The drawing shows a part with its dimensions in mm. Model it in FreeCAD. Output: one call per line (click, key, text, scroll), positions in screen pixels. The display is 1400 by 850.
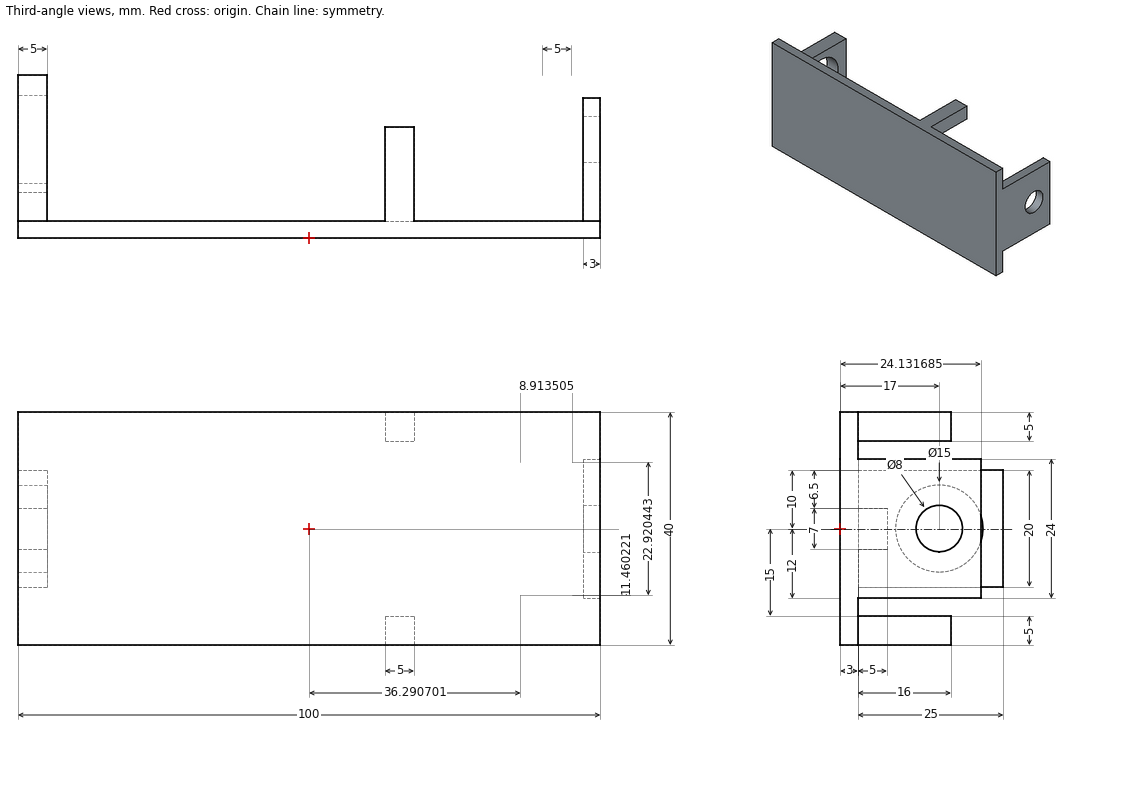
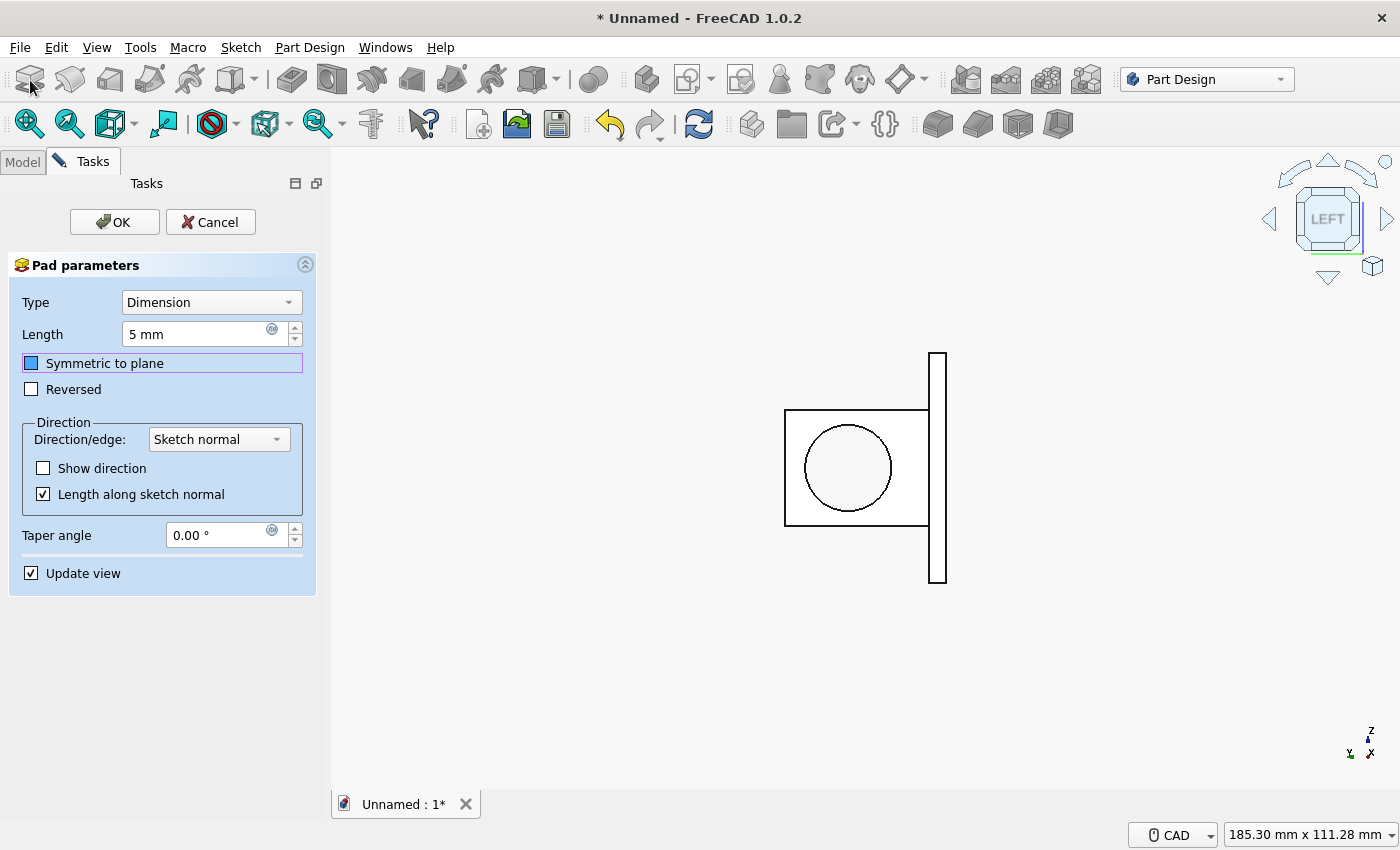
click(30, 389)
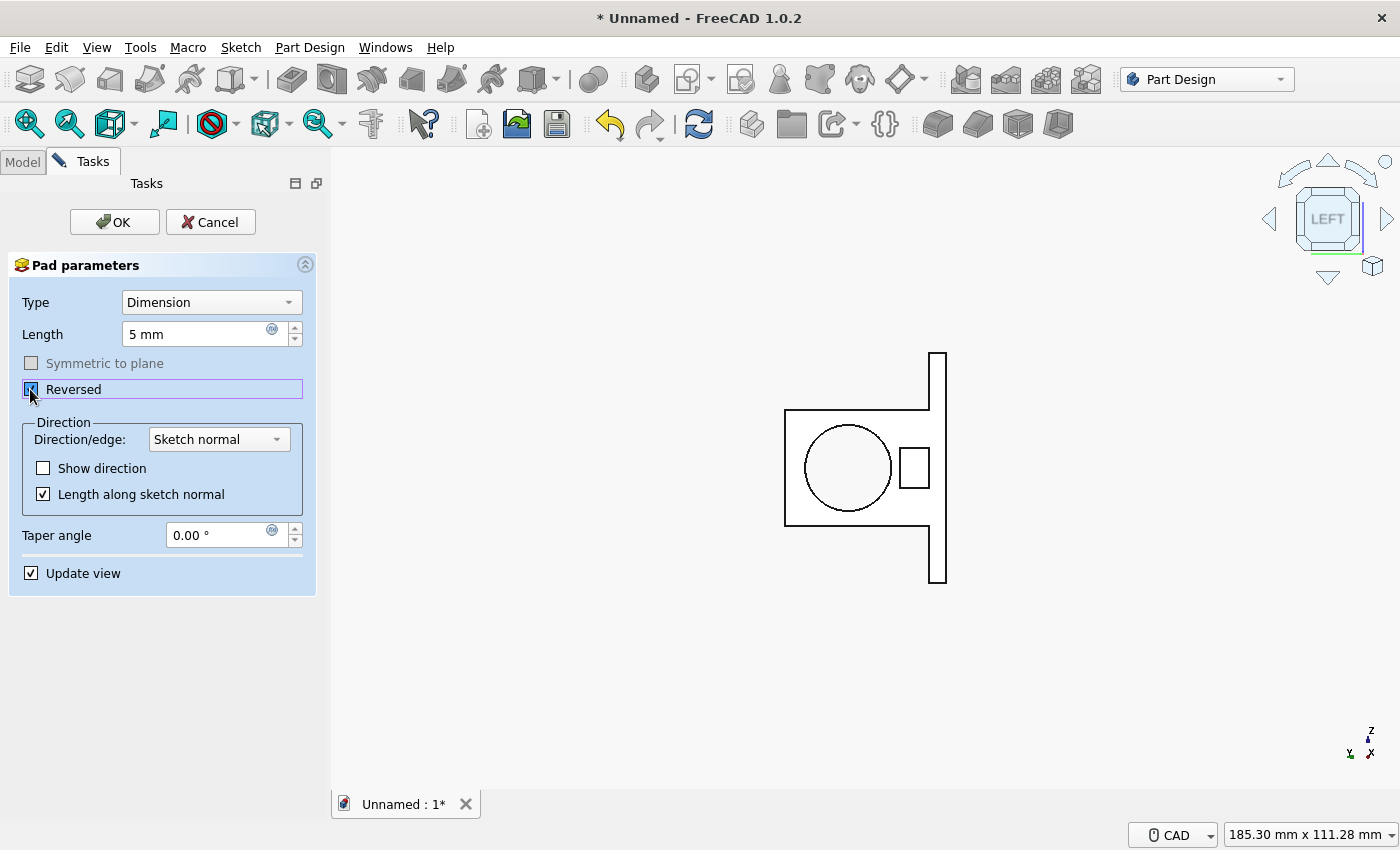
click(115, 222)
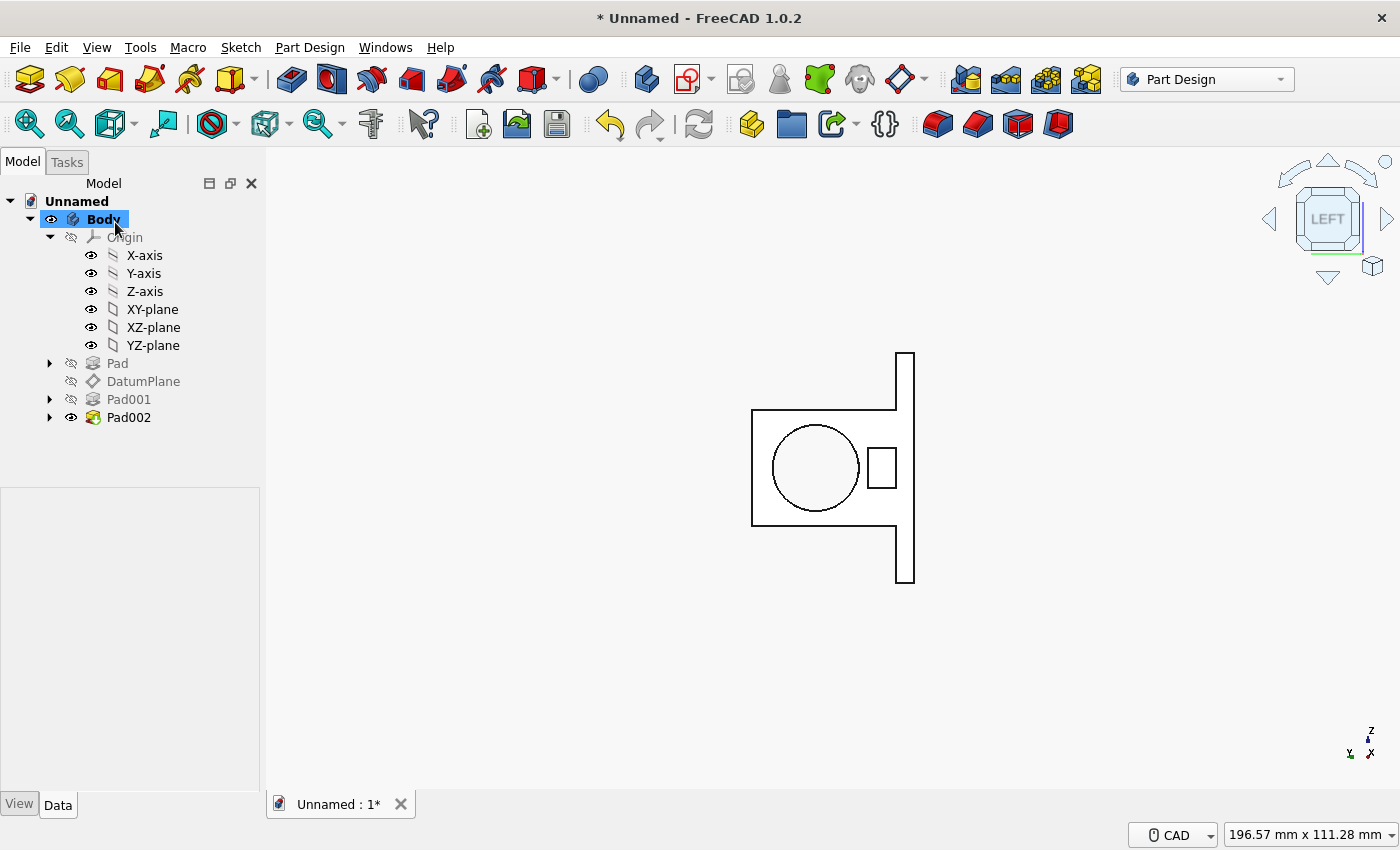
key(v)
key(f)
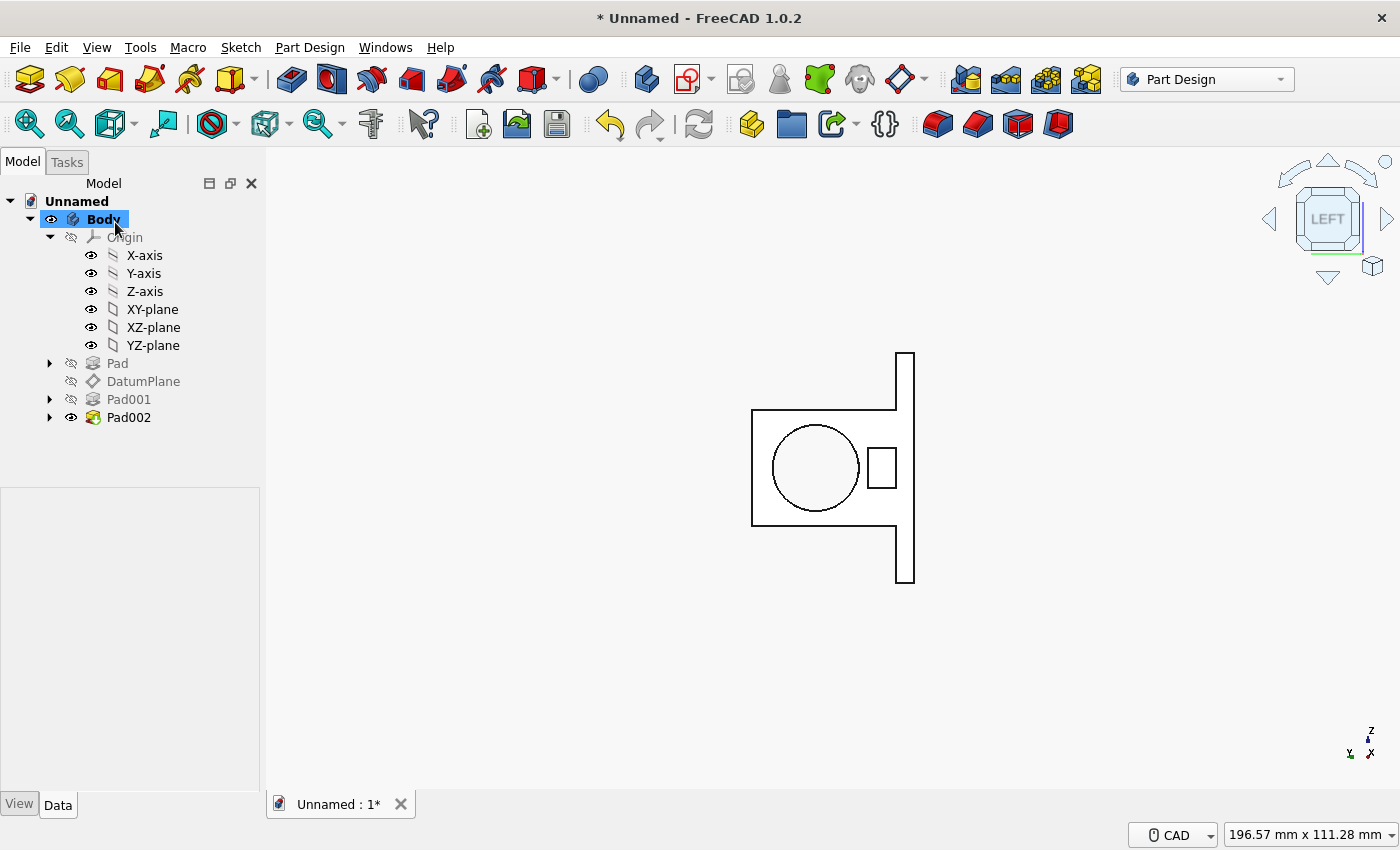
click(136, 345)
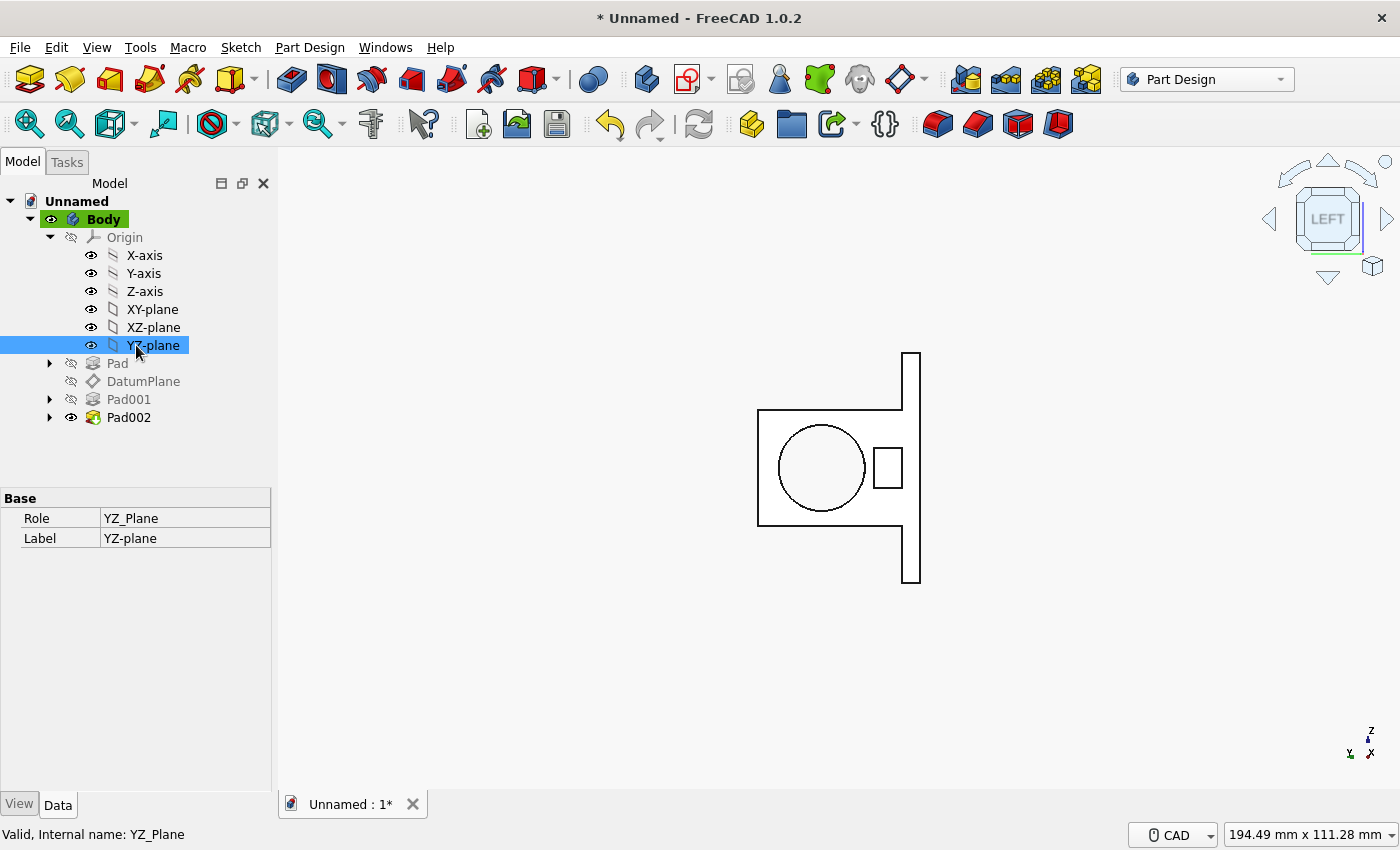
click(900, 80)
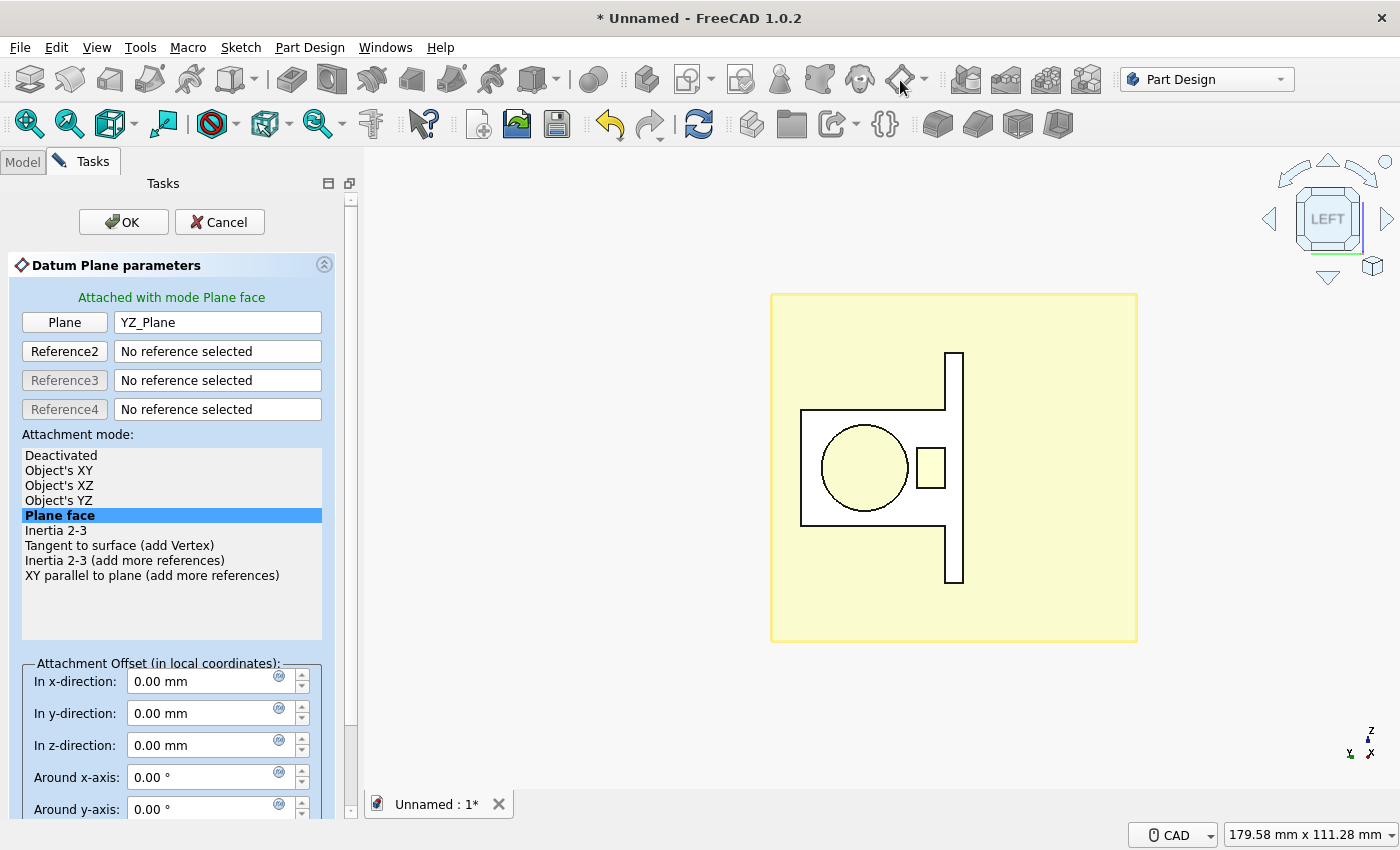
triple_click(210, 745)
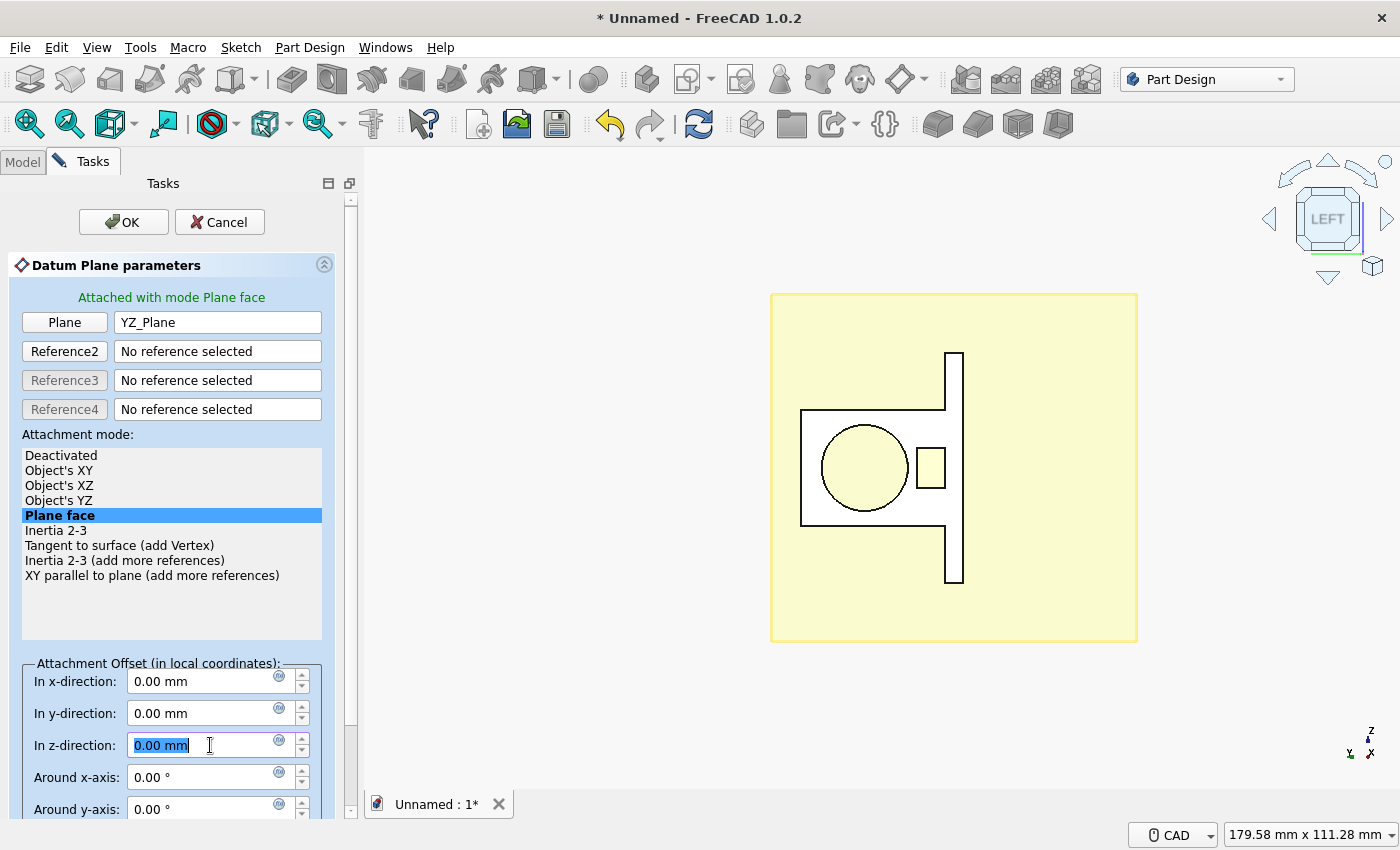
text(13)
key(Tab)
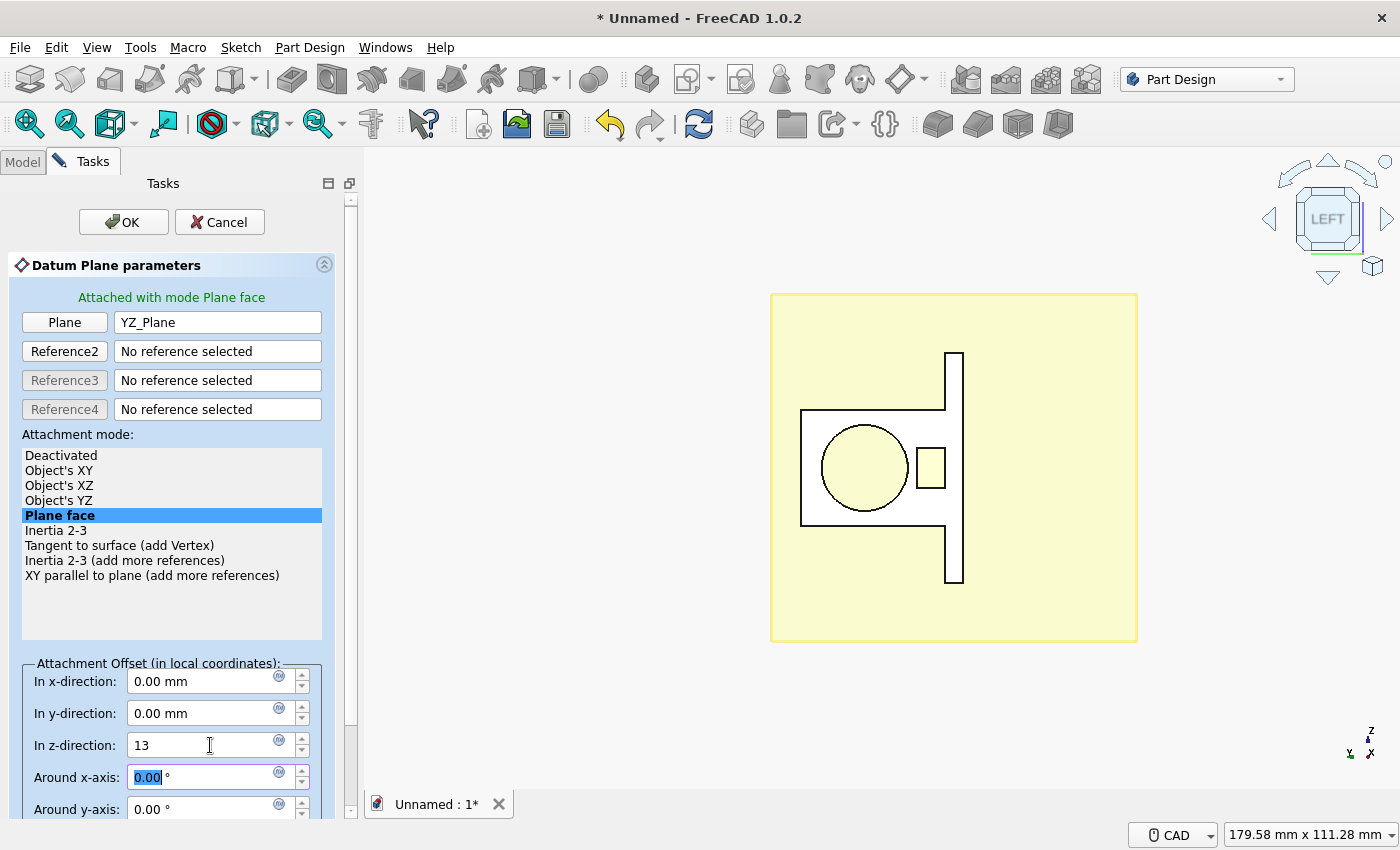
click(124, 222)